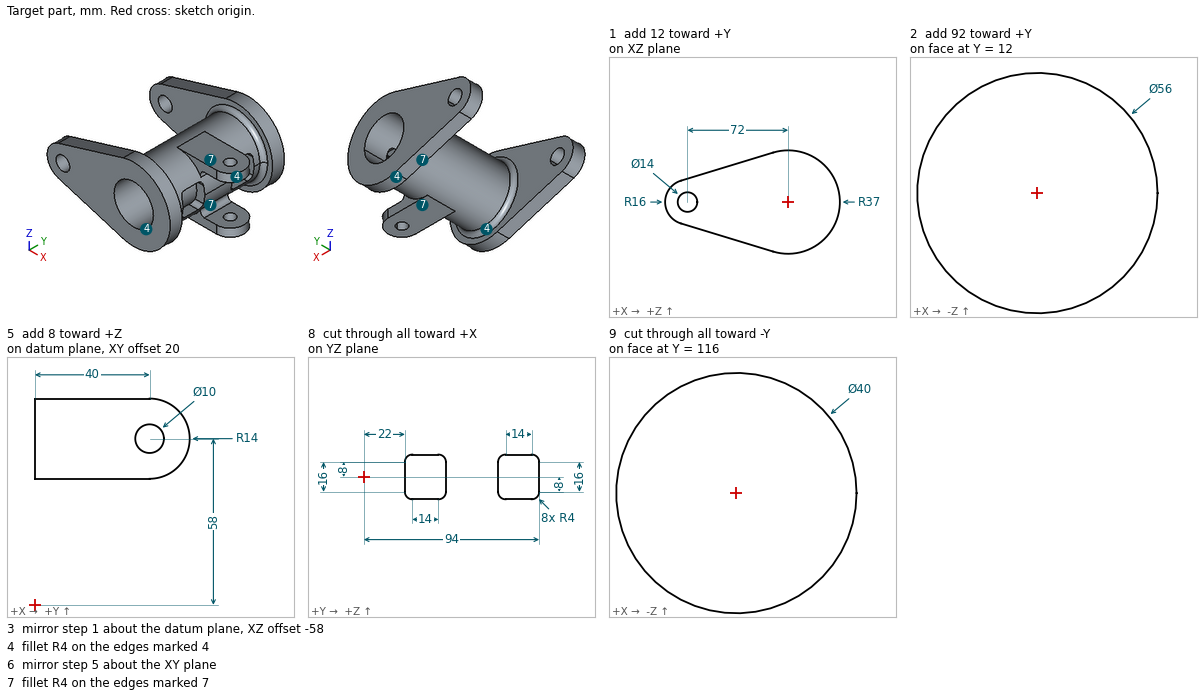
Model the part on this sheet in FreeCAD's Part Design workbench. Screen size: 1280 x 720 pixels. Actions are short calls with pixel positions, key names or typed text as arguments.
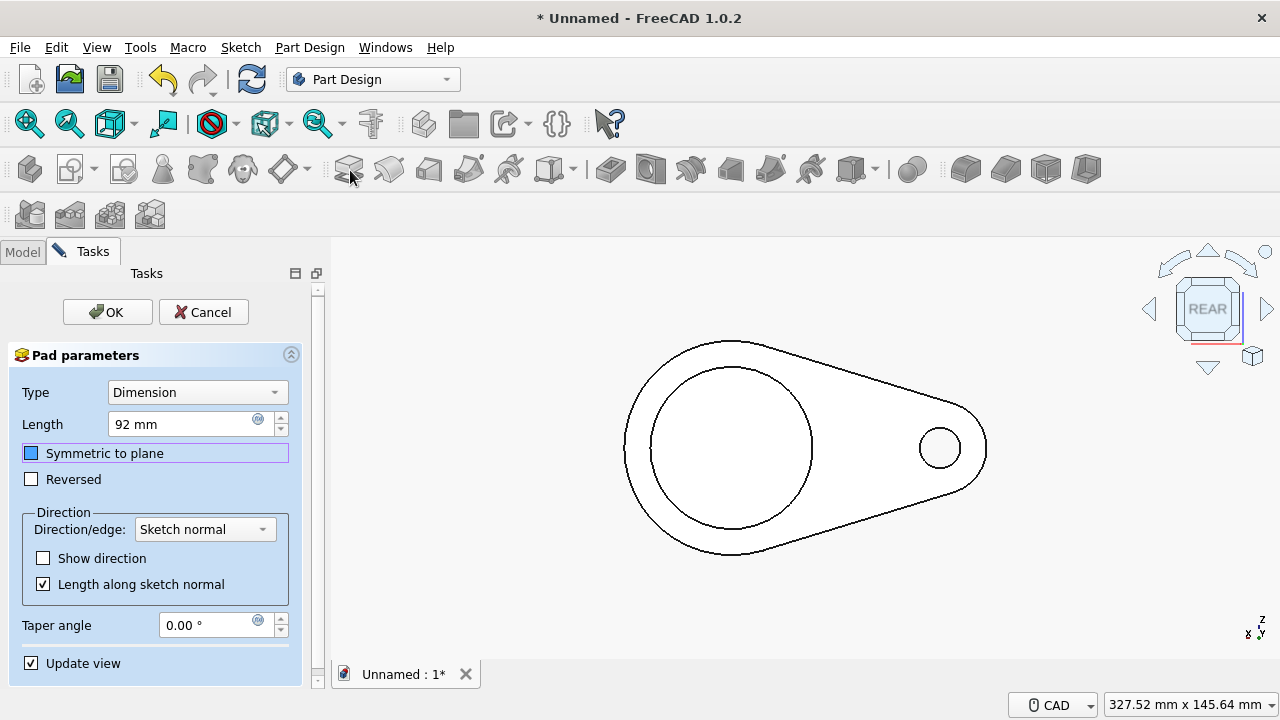
click(108, 312)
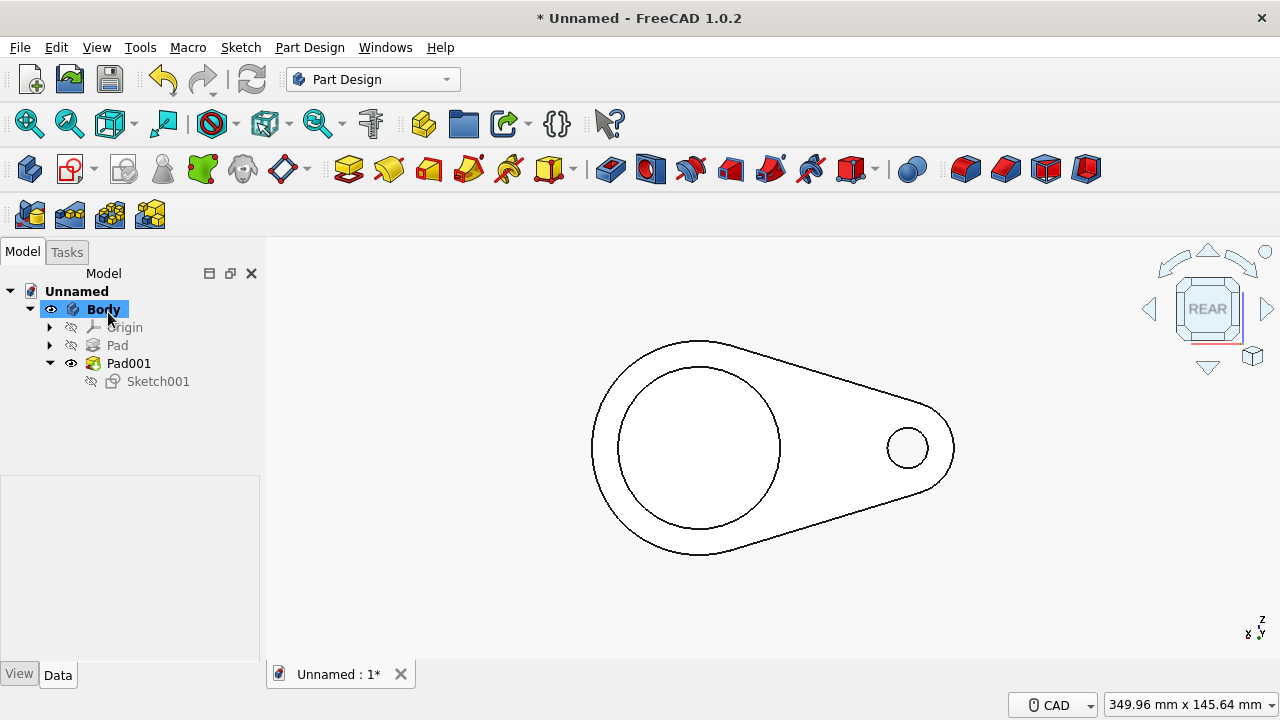
click(50, 327)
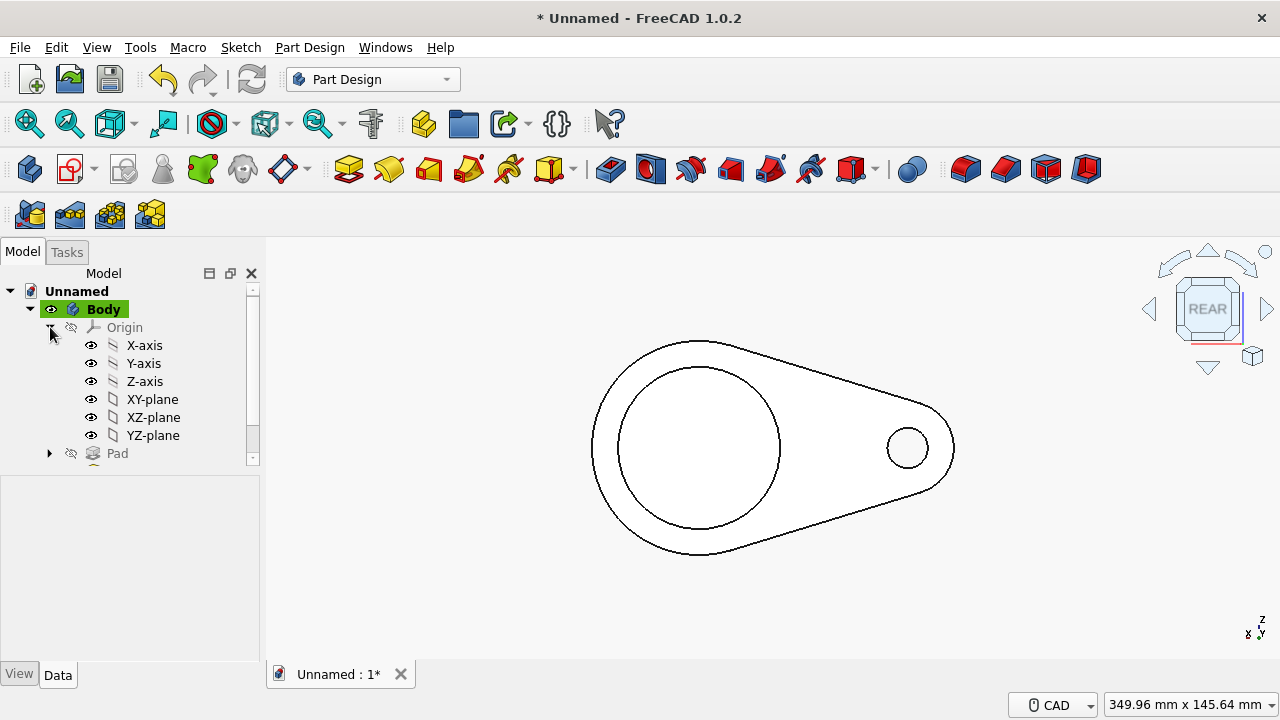
click(136, 417)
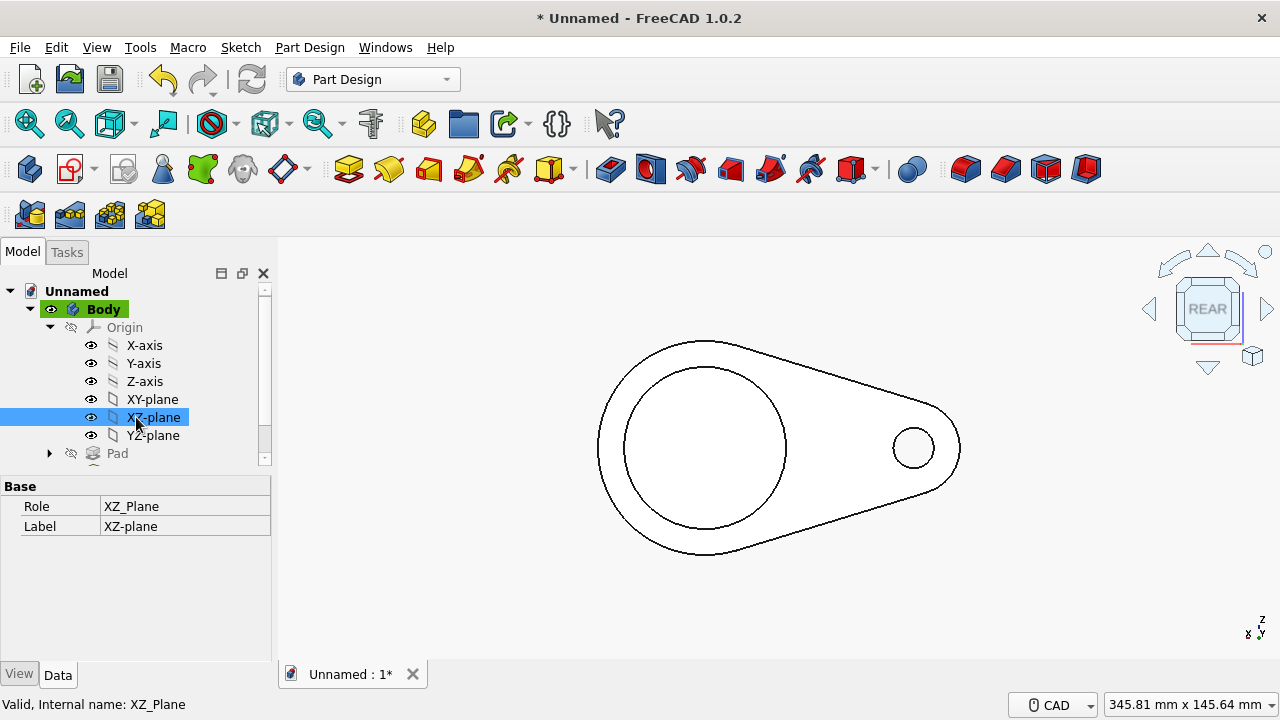
click(284, 170)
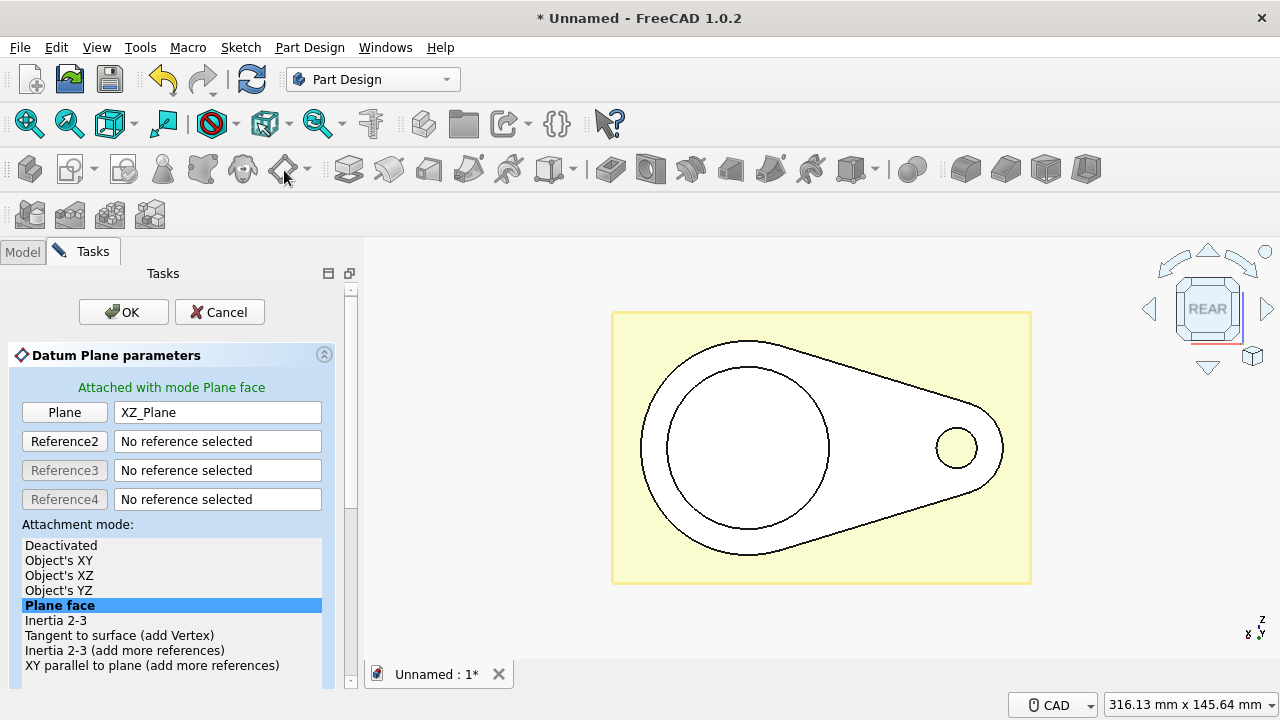
scroll(351, 486, down, 4)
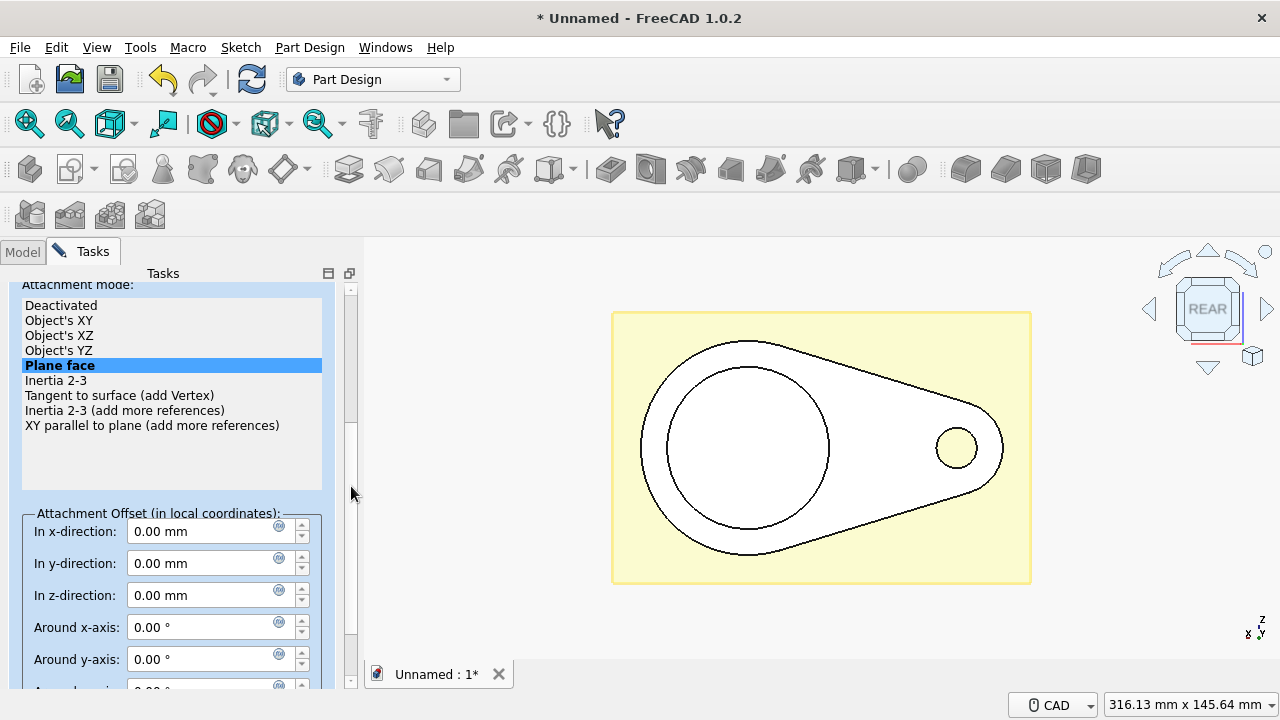
triple_click(210, 595)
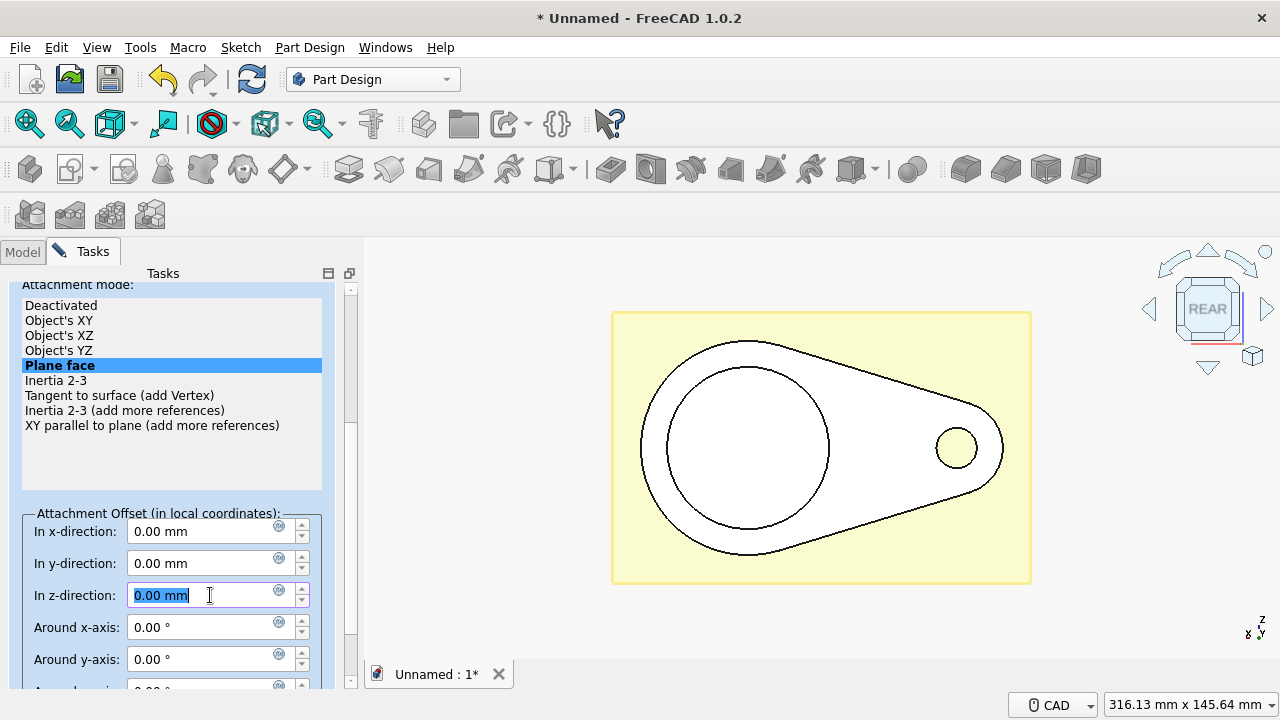
text(-58)
key(Tab)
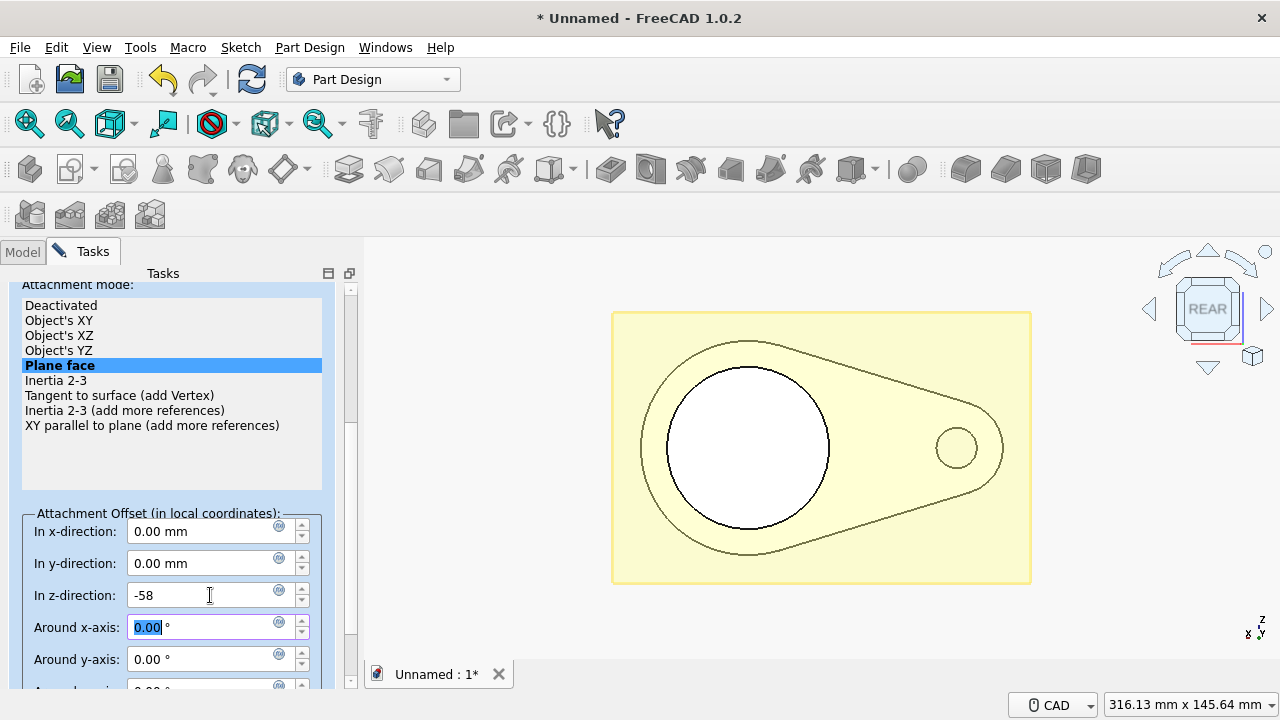
scroll(351, 486, up, 5)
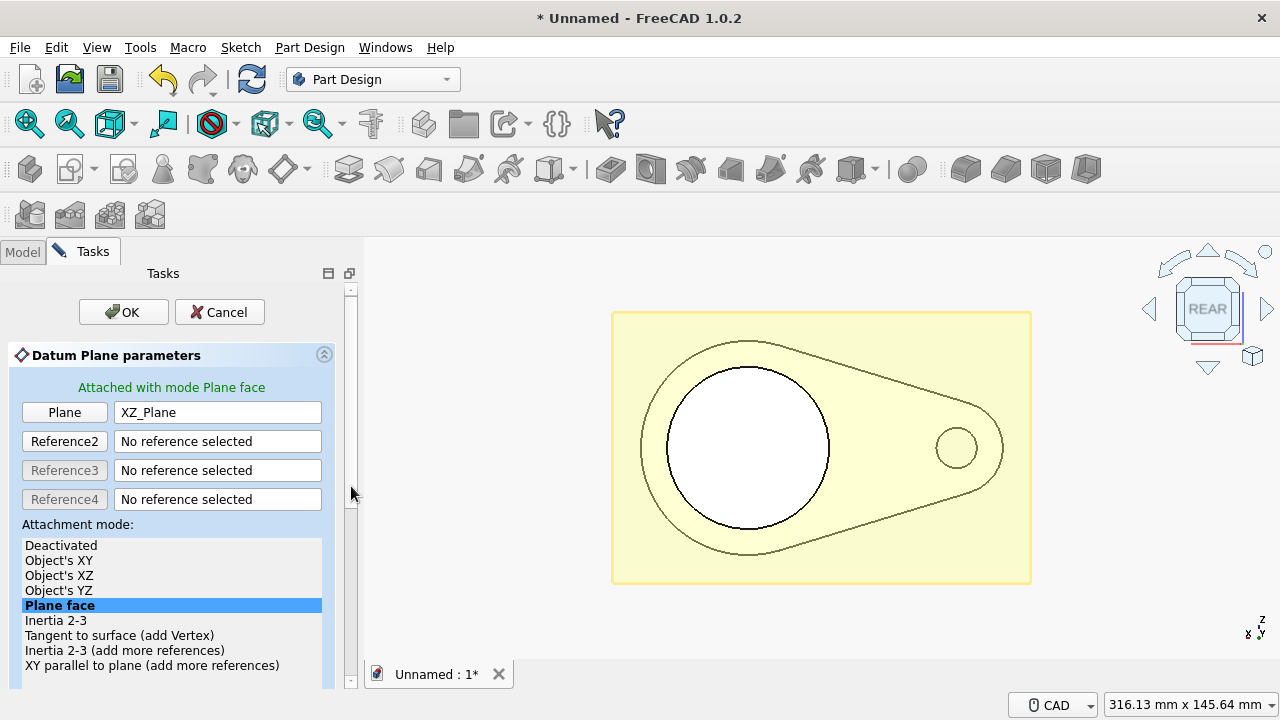
click(124, 312)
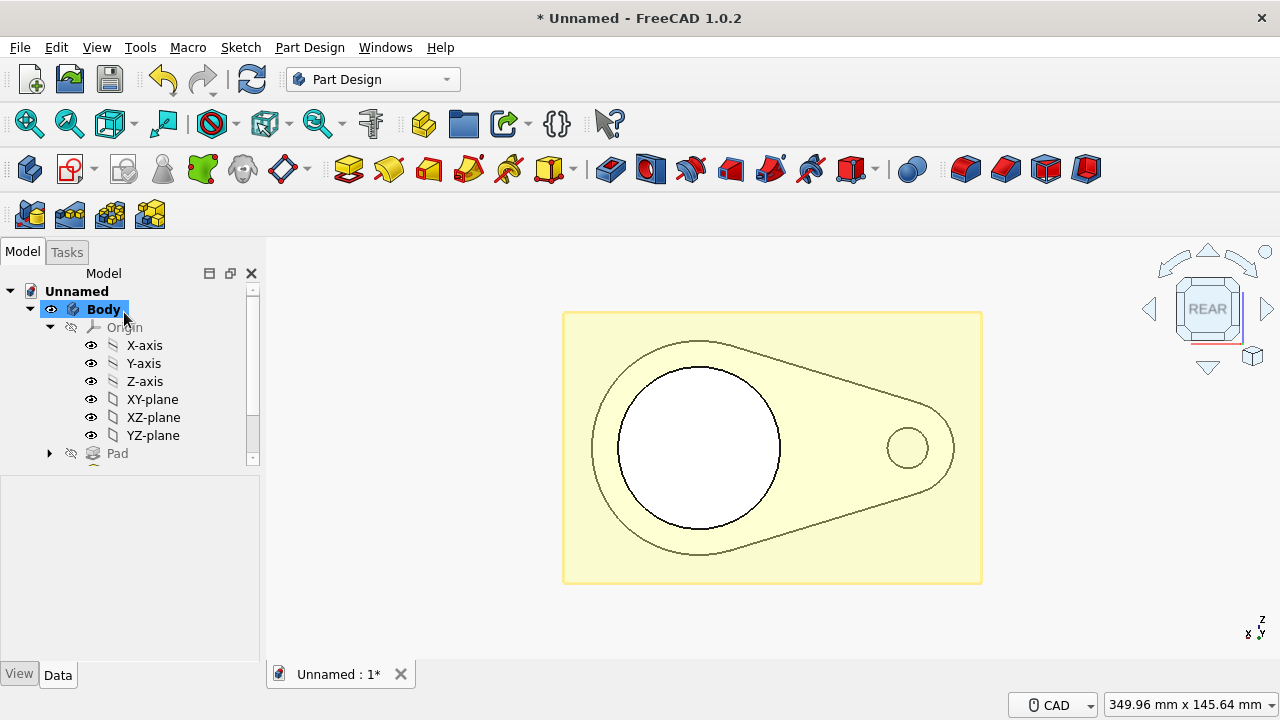
click(116, 453)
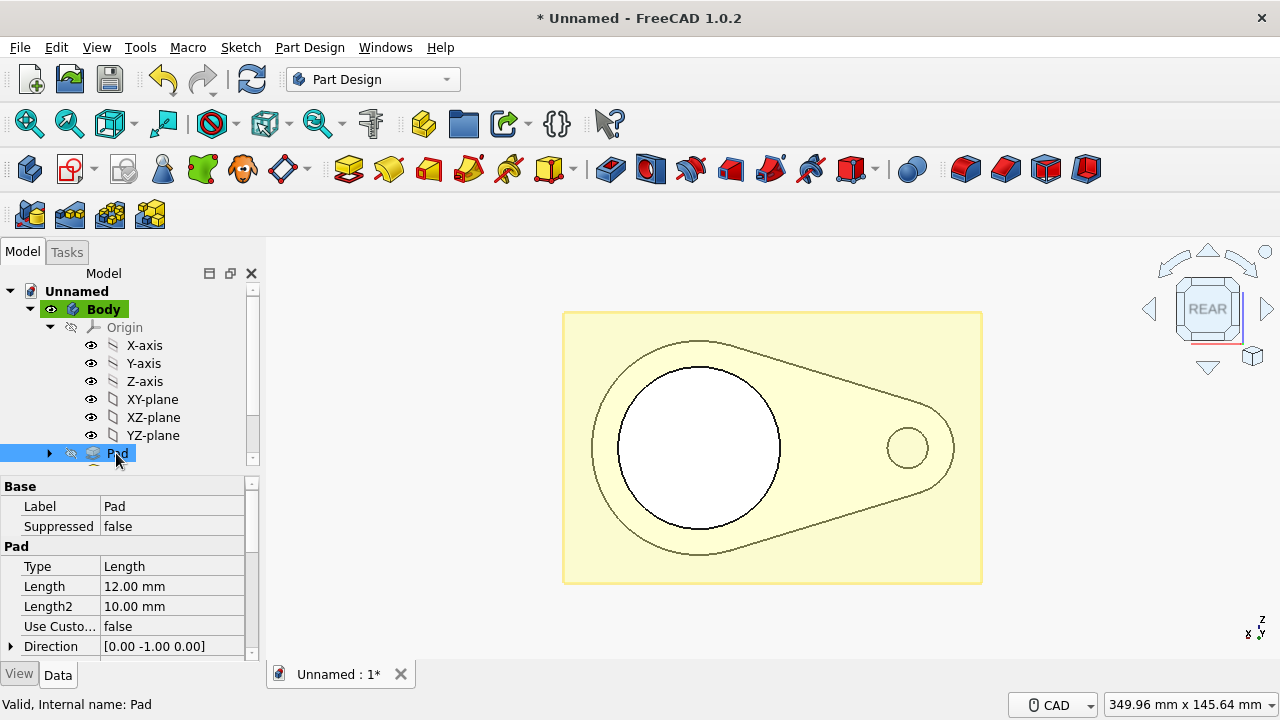
click(30, 214)